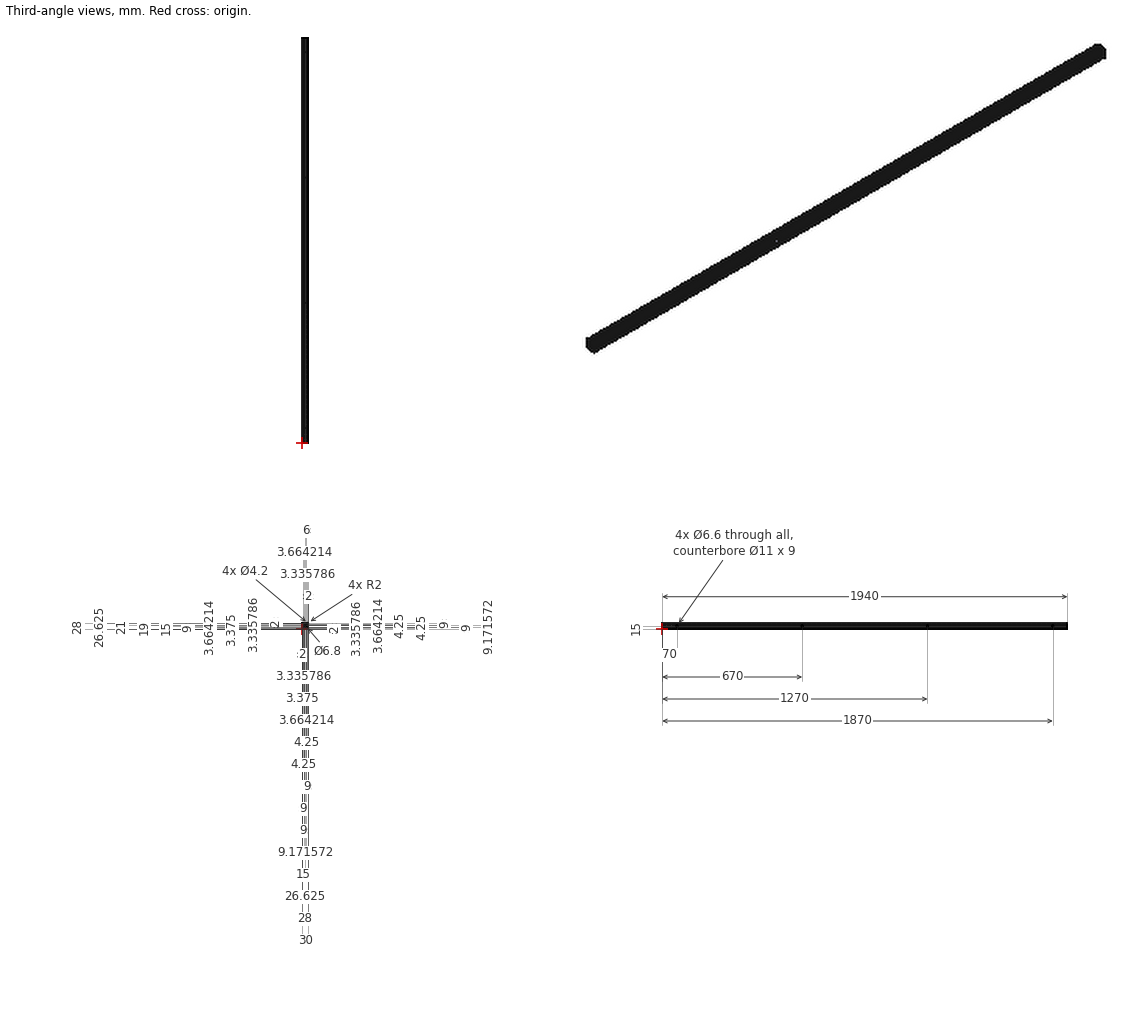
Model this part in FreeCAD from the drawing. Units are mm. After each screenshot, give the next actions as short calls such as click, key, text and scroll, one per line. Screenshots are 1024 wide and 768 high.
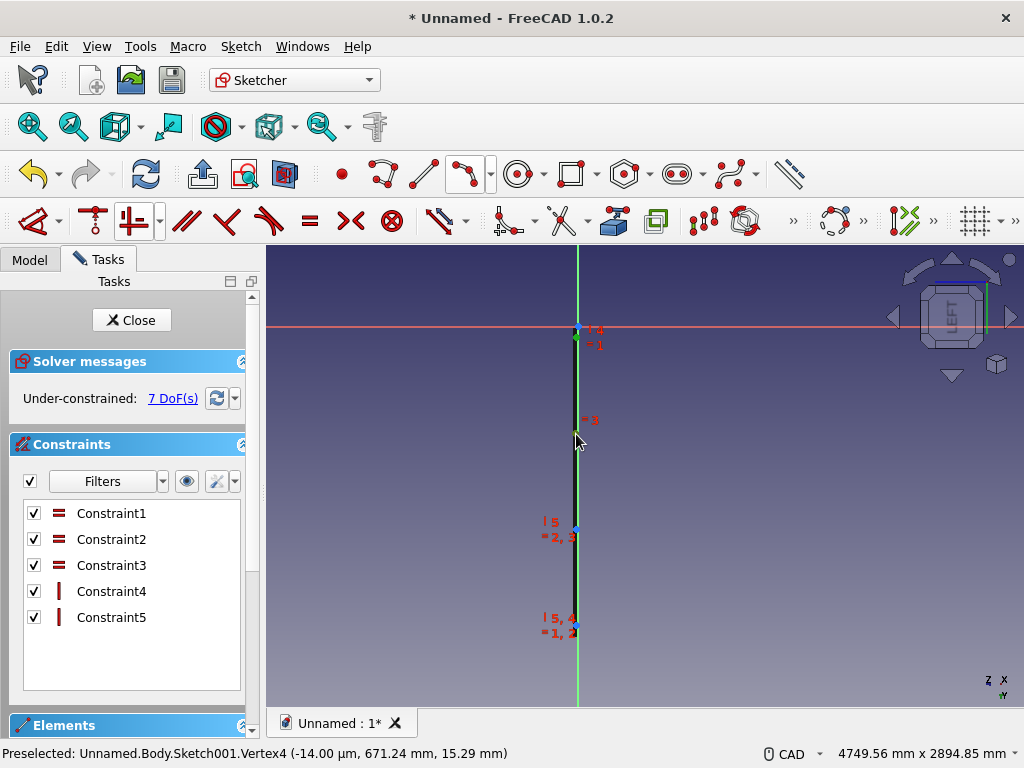
click(160, 222)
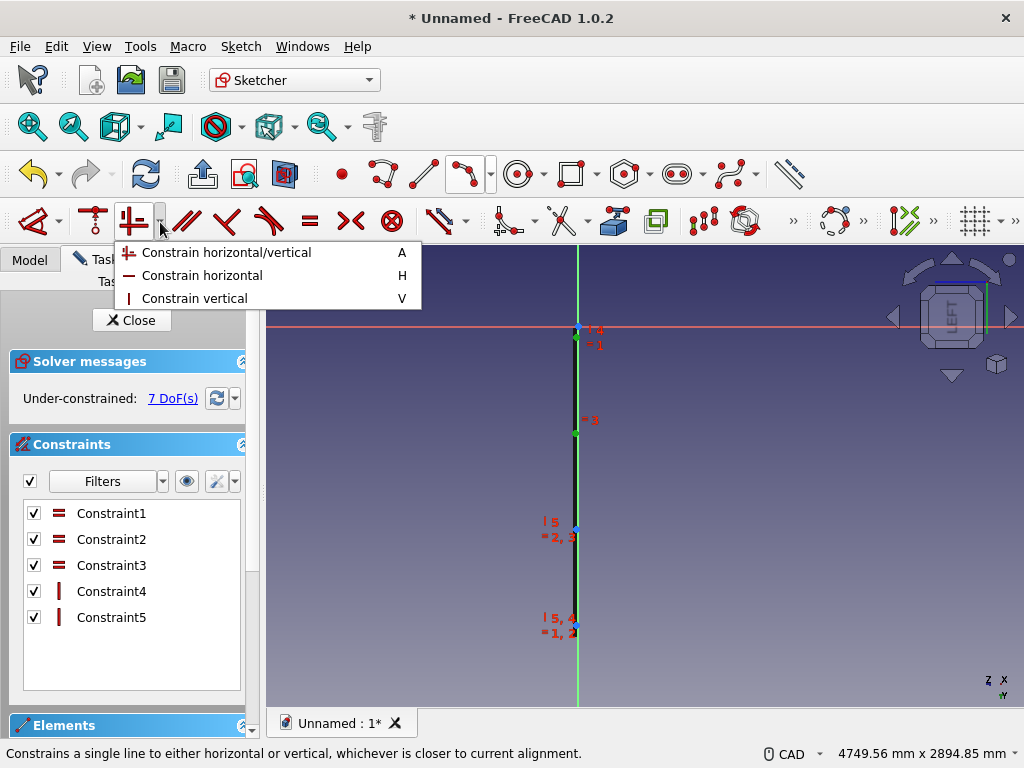
click(268, 298)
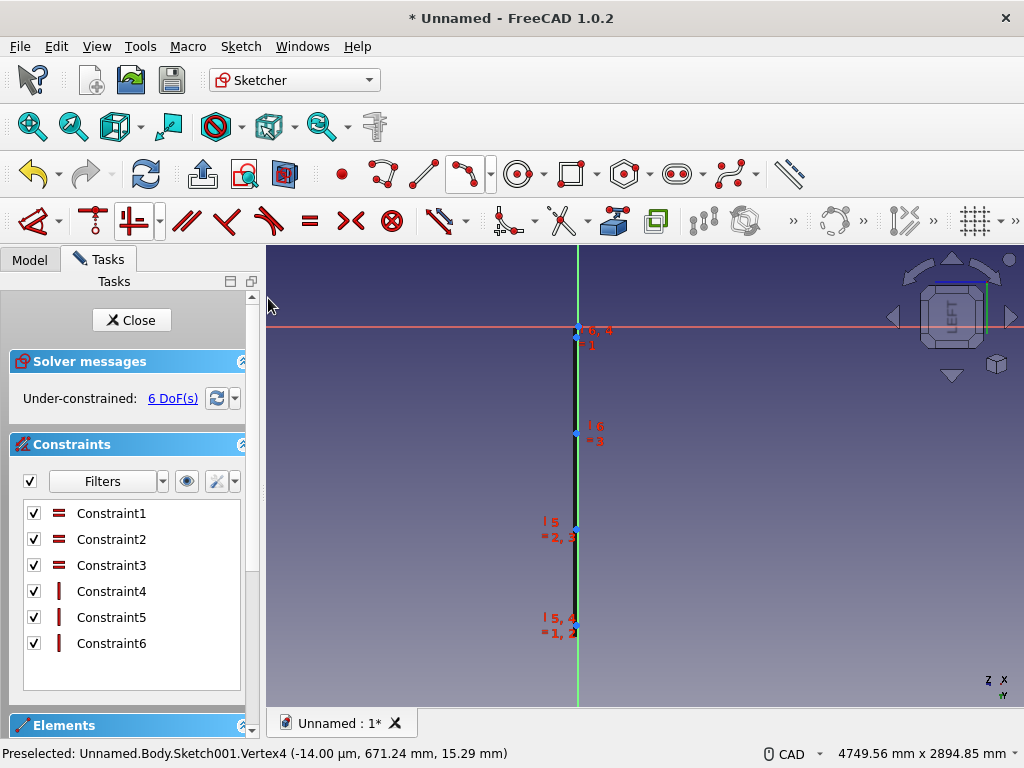
key(d)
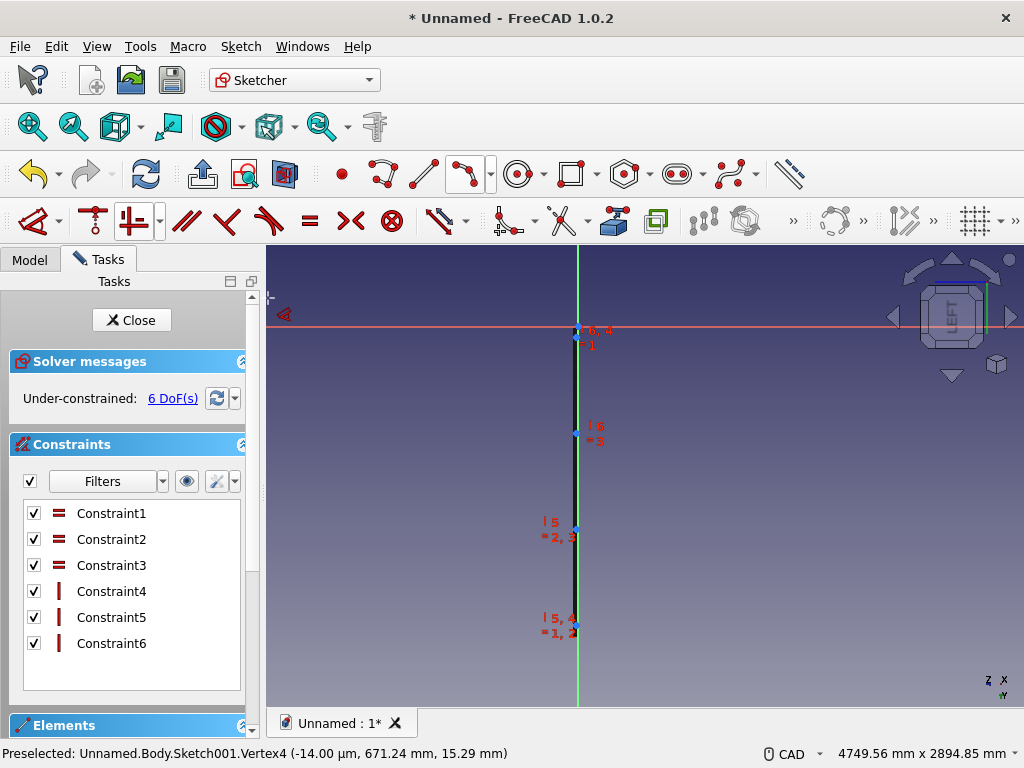
scroll(576, 337, up, 19)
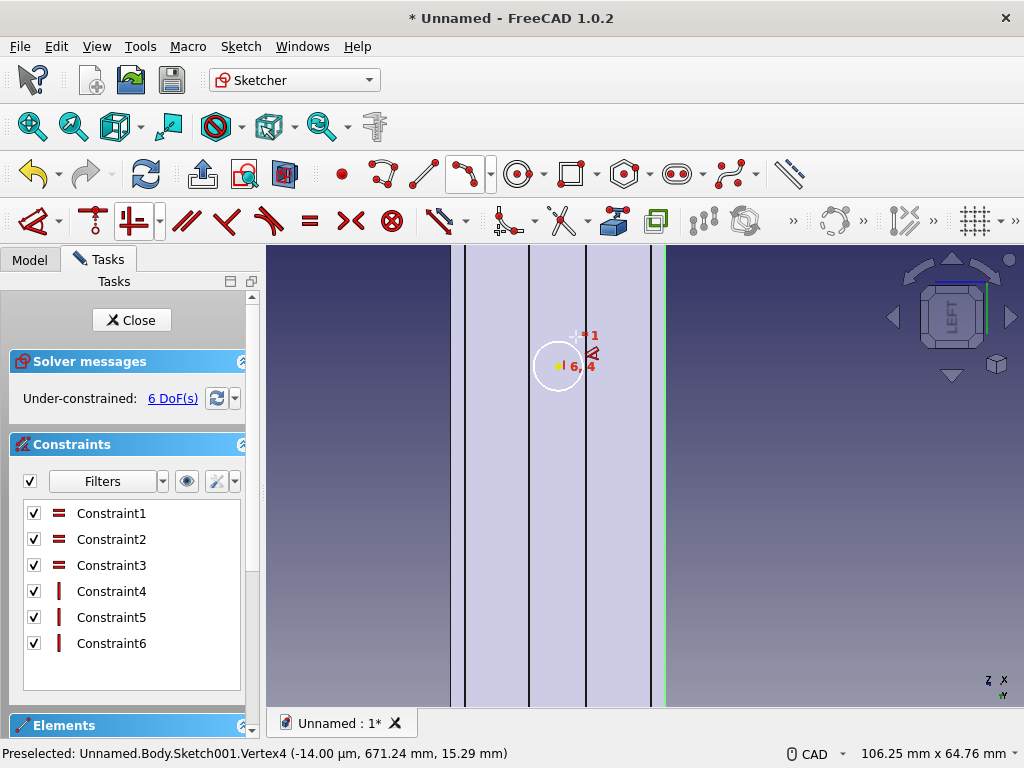
click(541, 349)
click(518, 326)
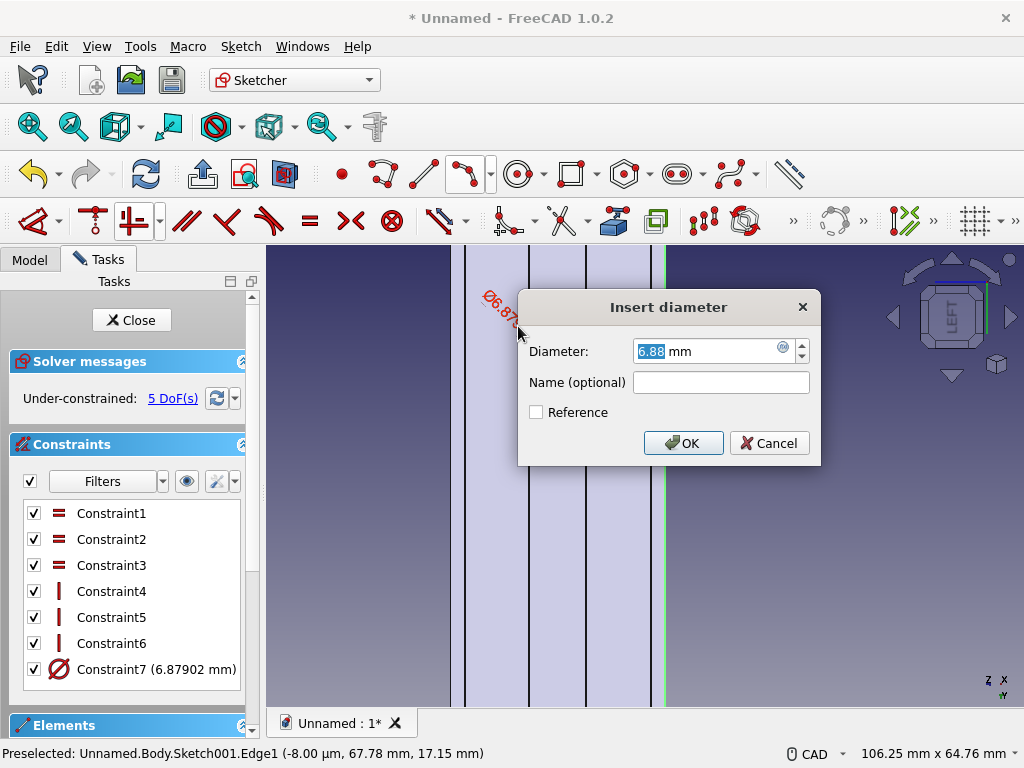
text(6.6)
key(Return)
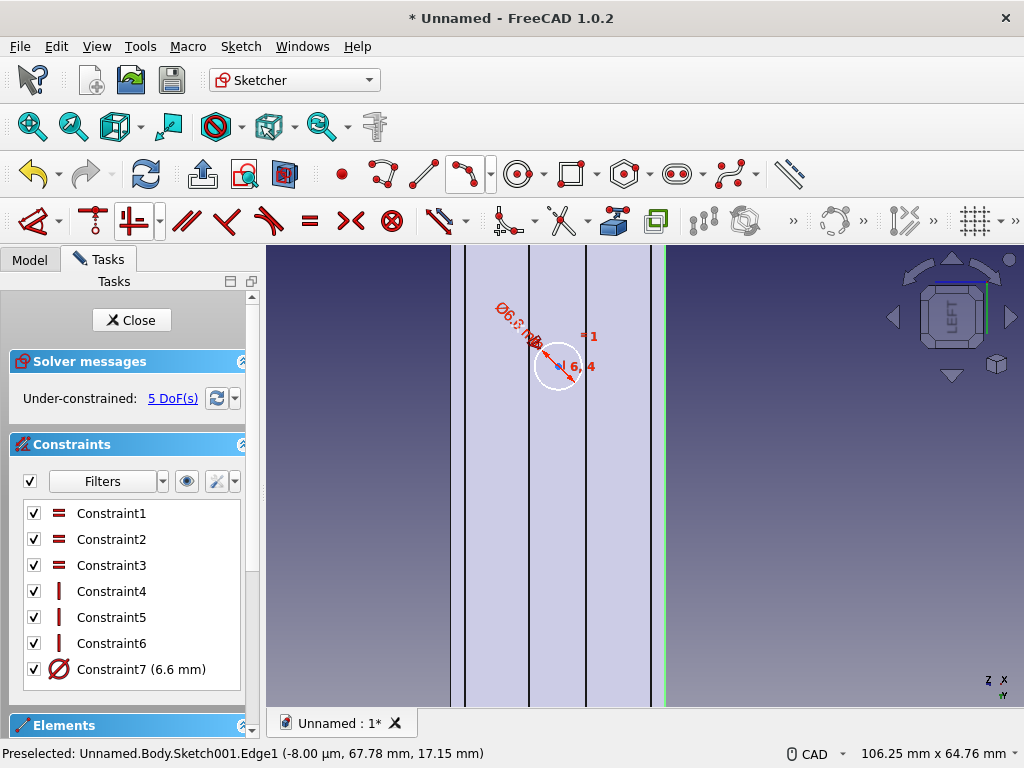
click(558, 366)
click(612, 400)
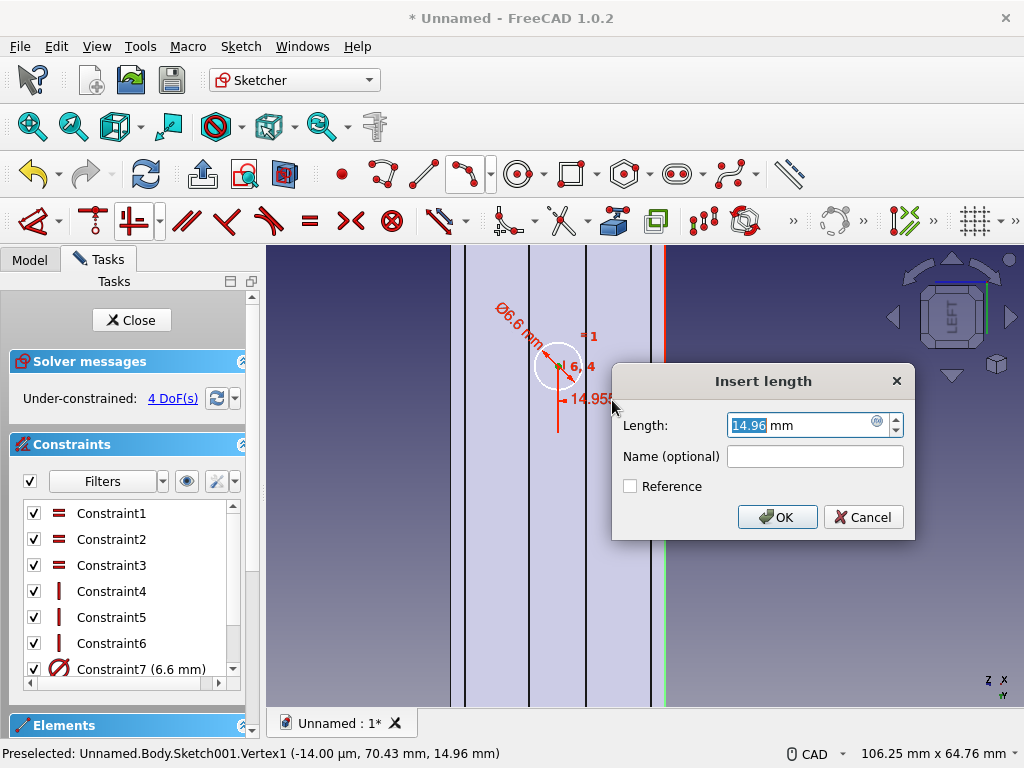
text(15)
key(Return)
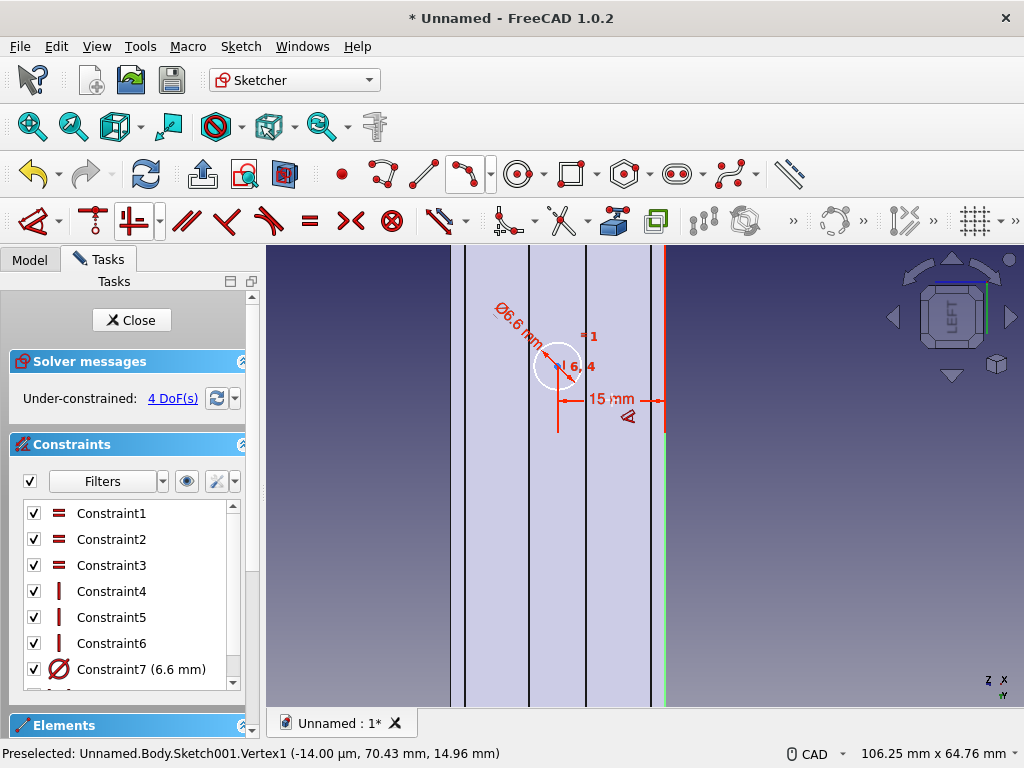
scroll(576, 476, down, 15)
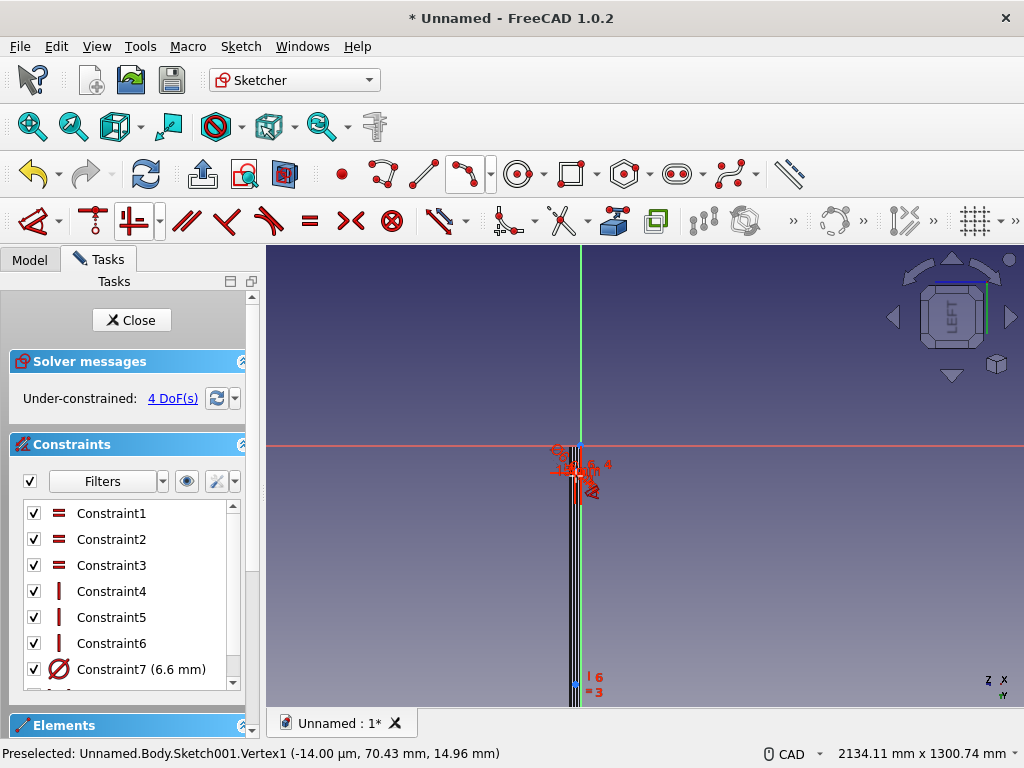
scroll(576, 273, down, 4)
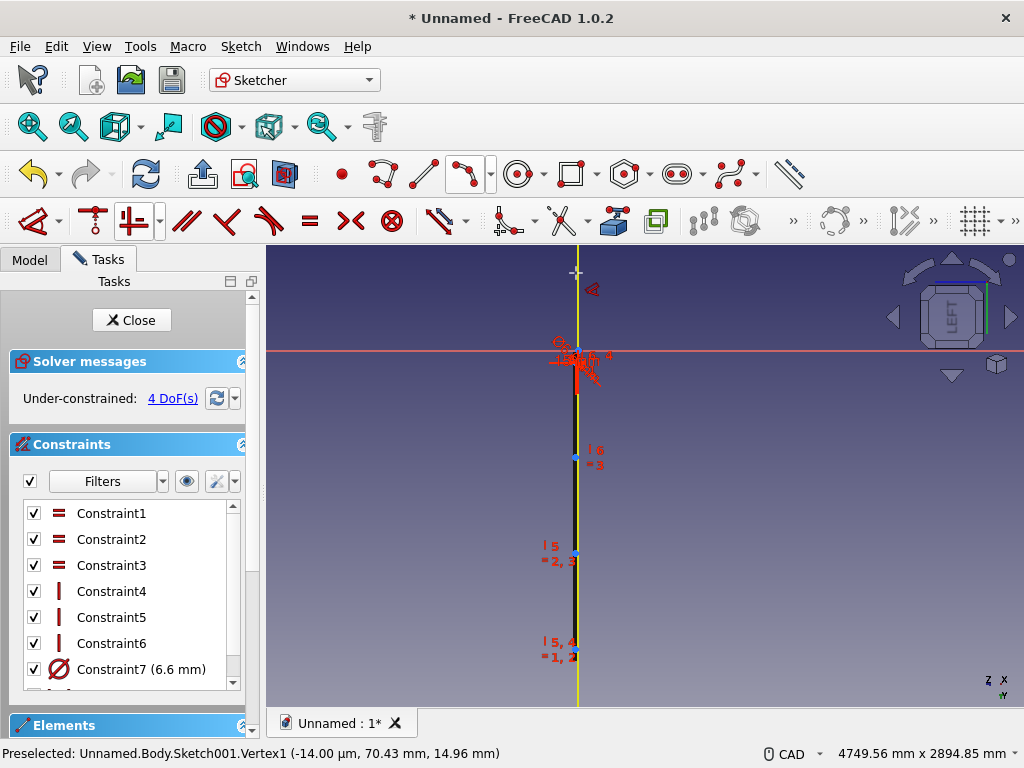
scroll(576, 362, up, 7)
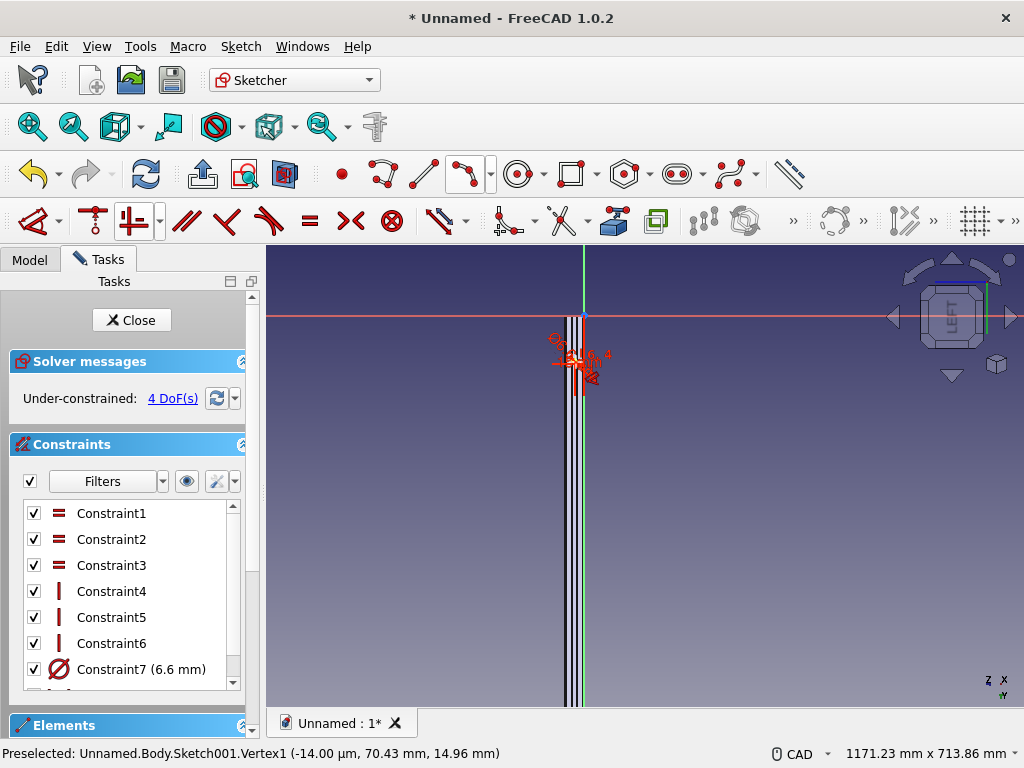
click(575, 361)
click(642, 338)